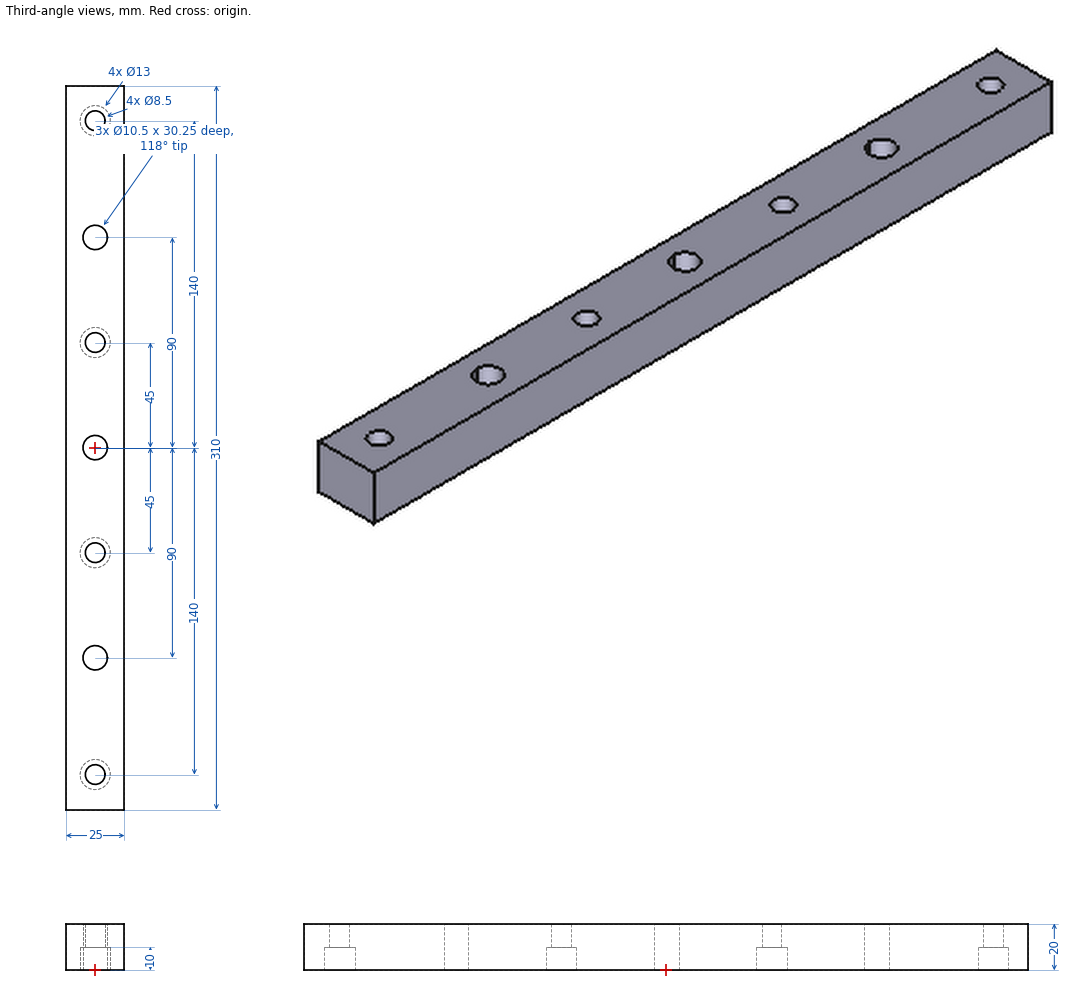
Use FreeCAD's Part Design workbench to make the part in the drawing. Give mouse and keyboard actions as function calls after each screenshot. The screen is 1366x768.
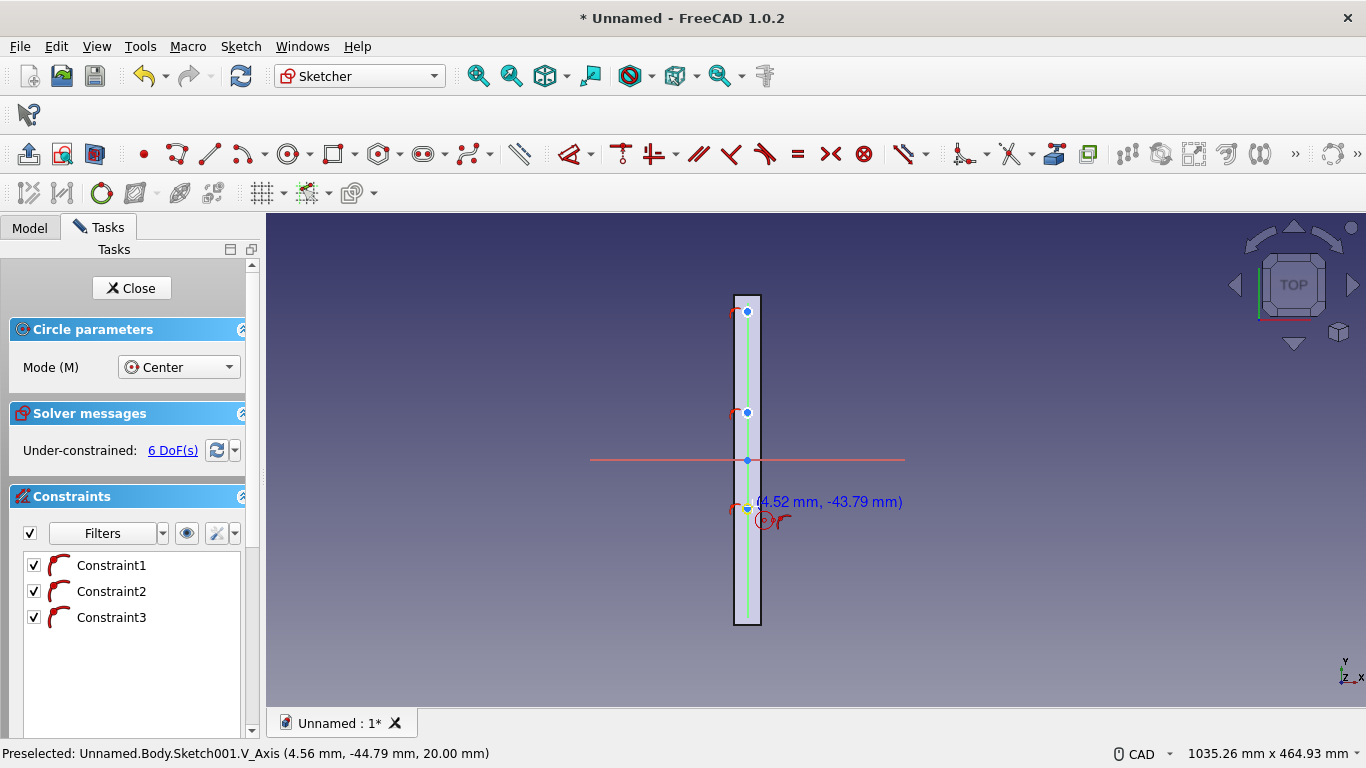
scroll(748, 609, up, 9)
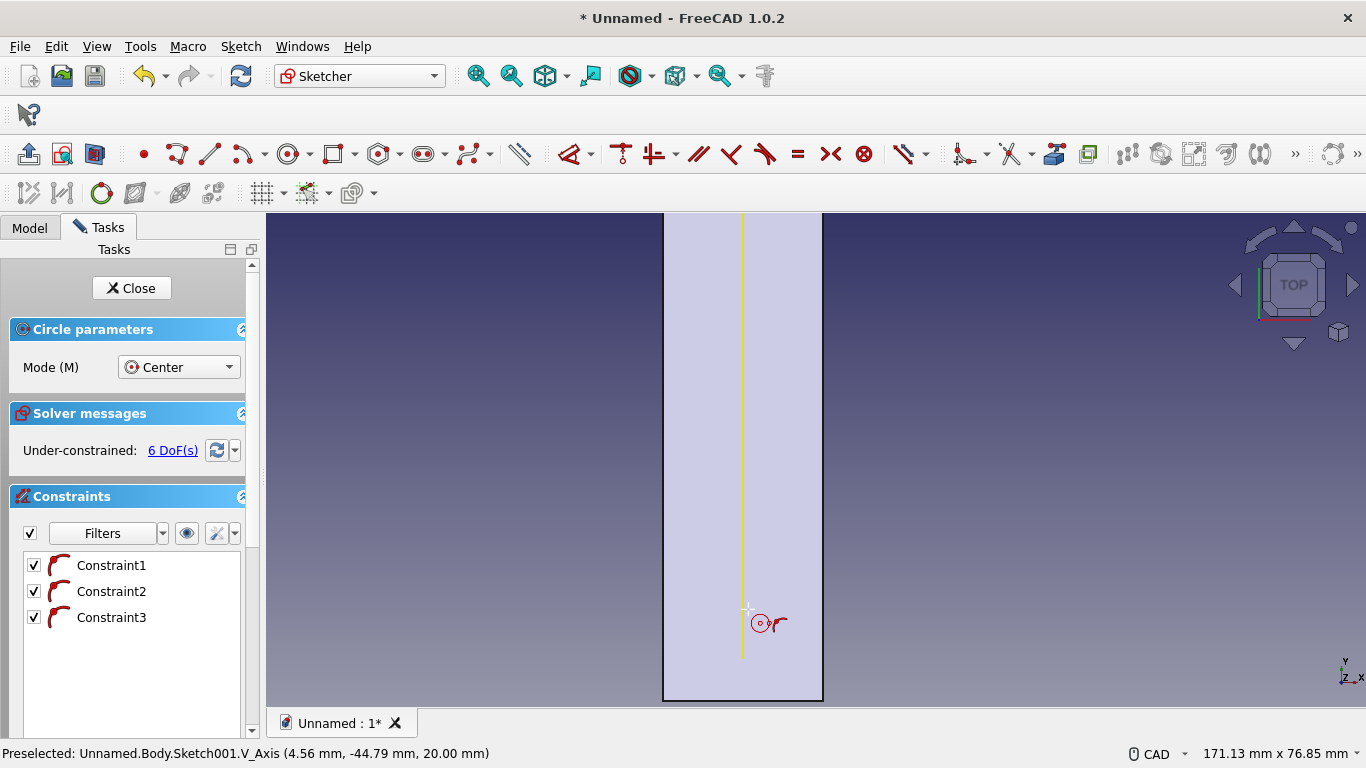
scroll(748, 610, down, 9)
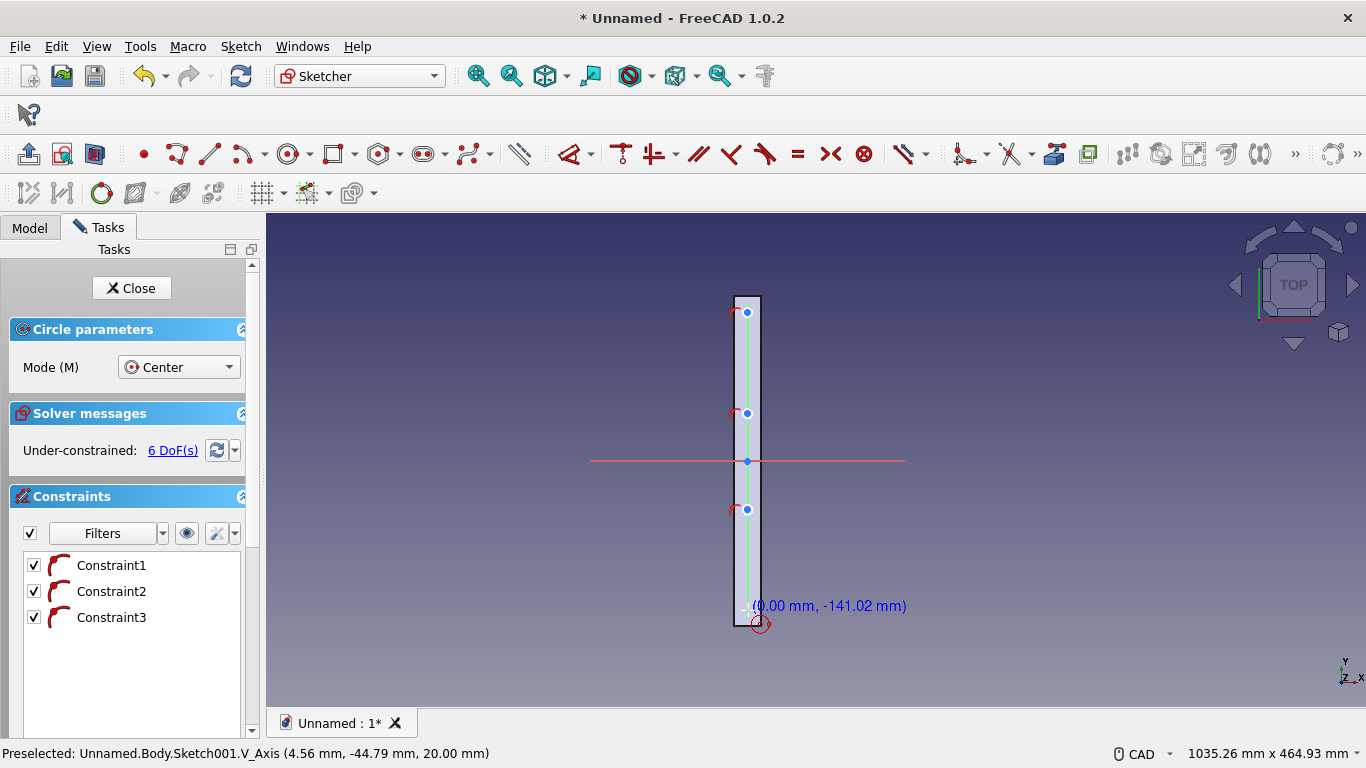
click(748, 610)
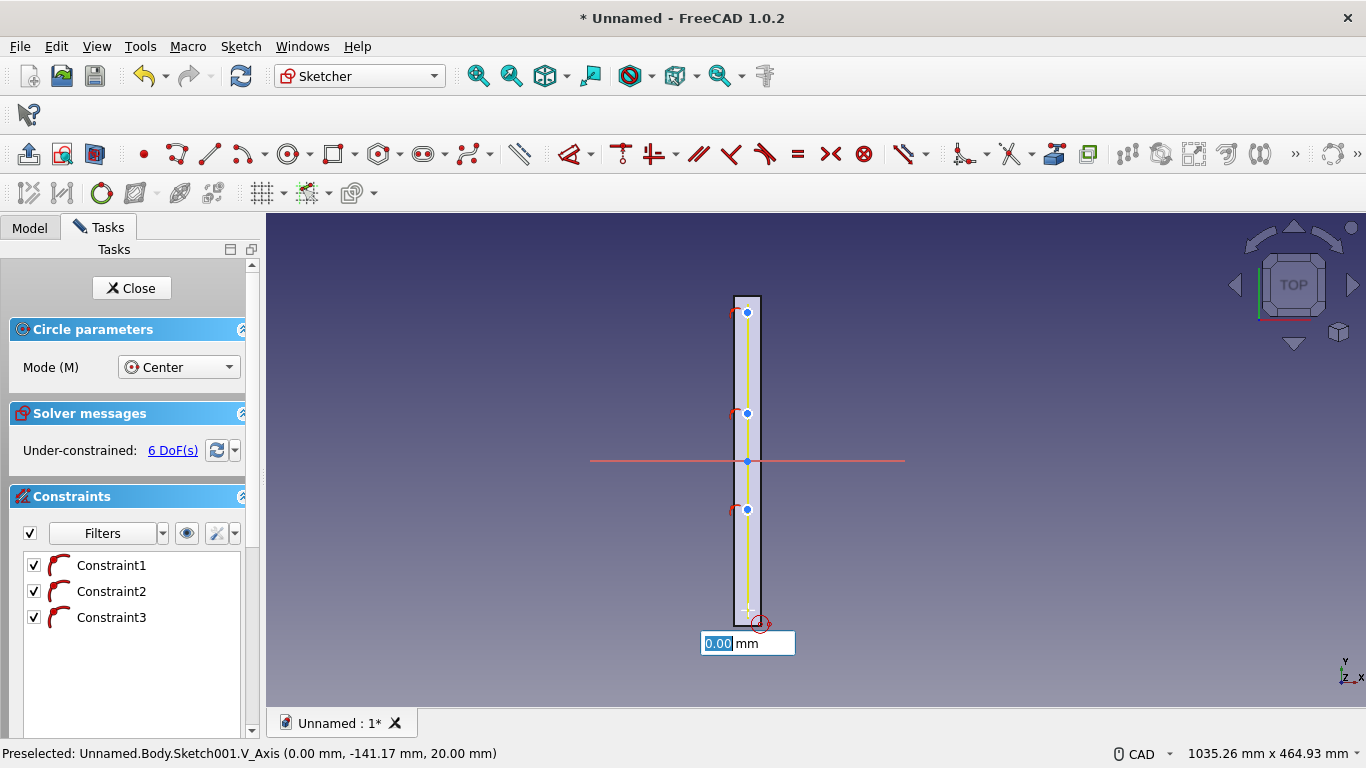
scroll(752, 608, up, 7)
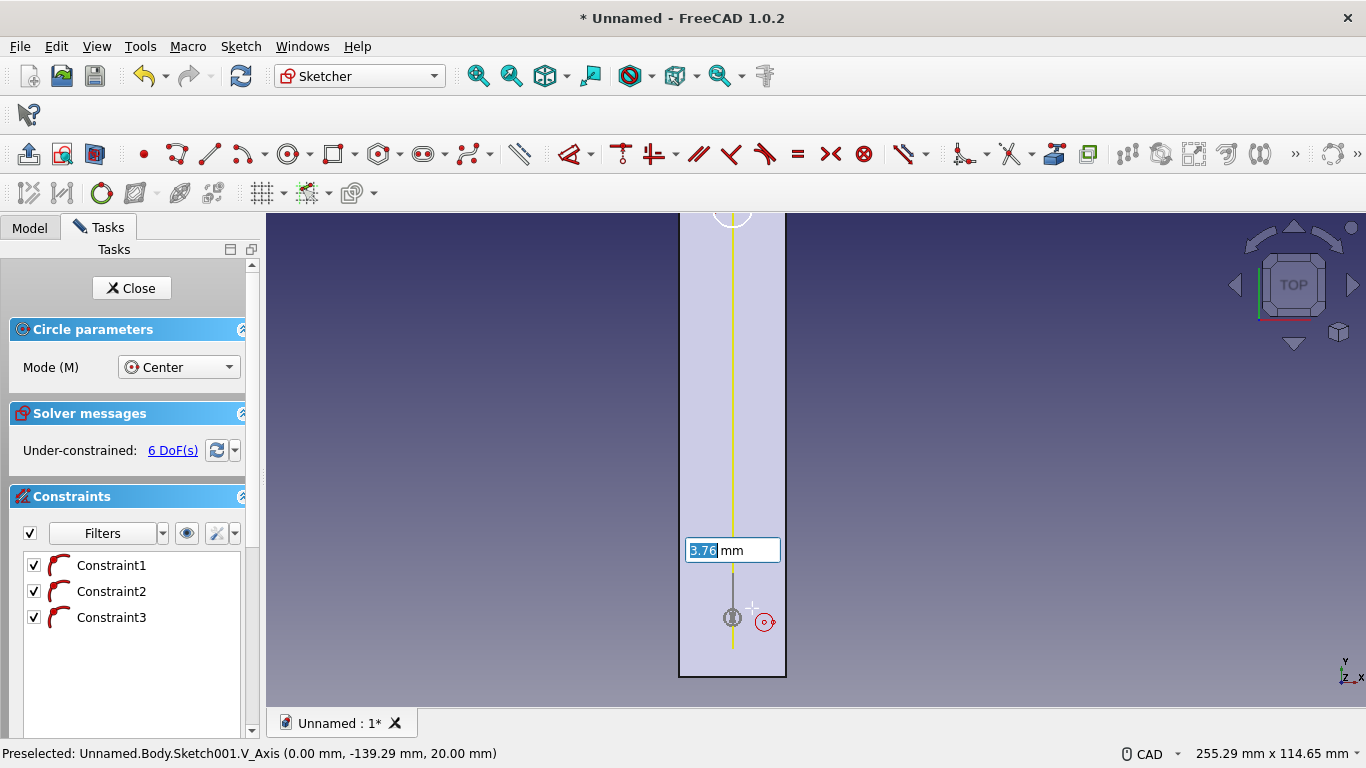
click(750, 606)
key(Escape)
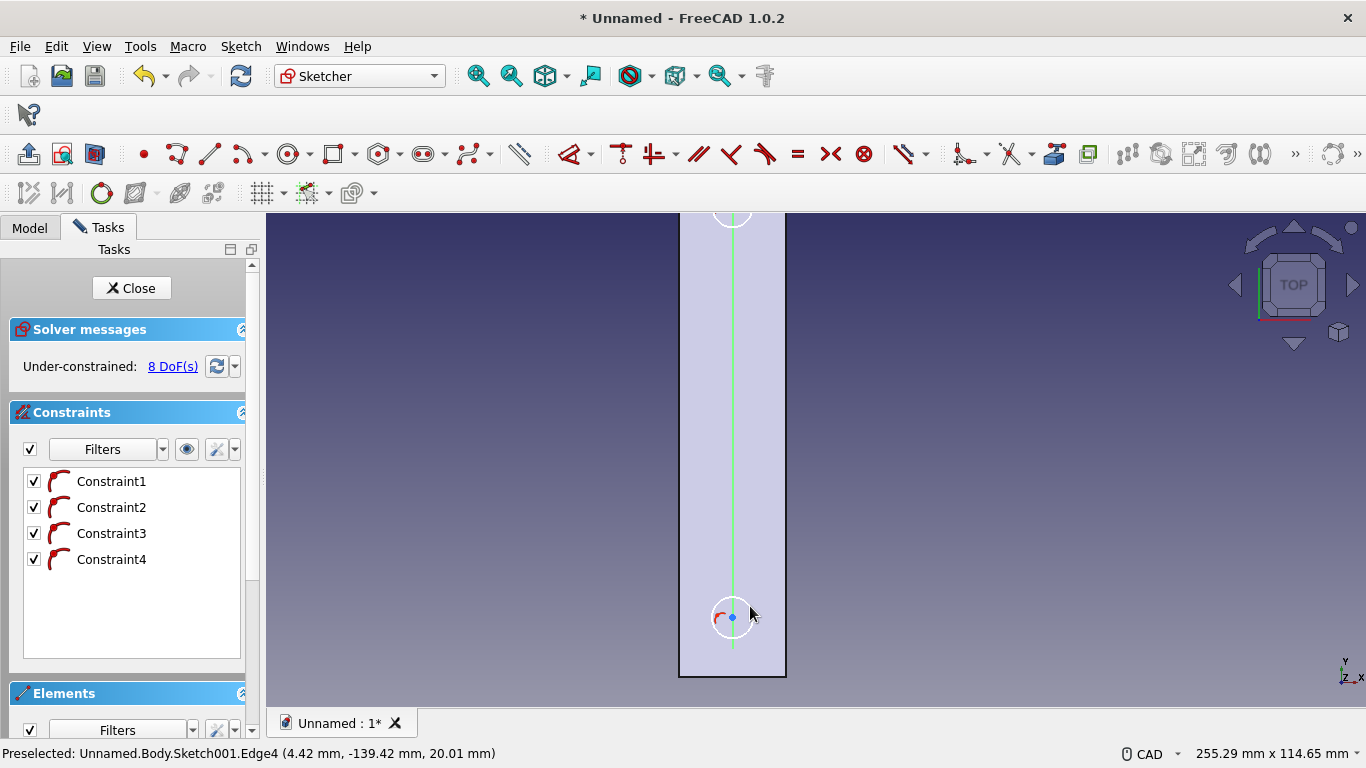
scroll(752, 607, down, 7)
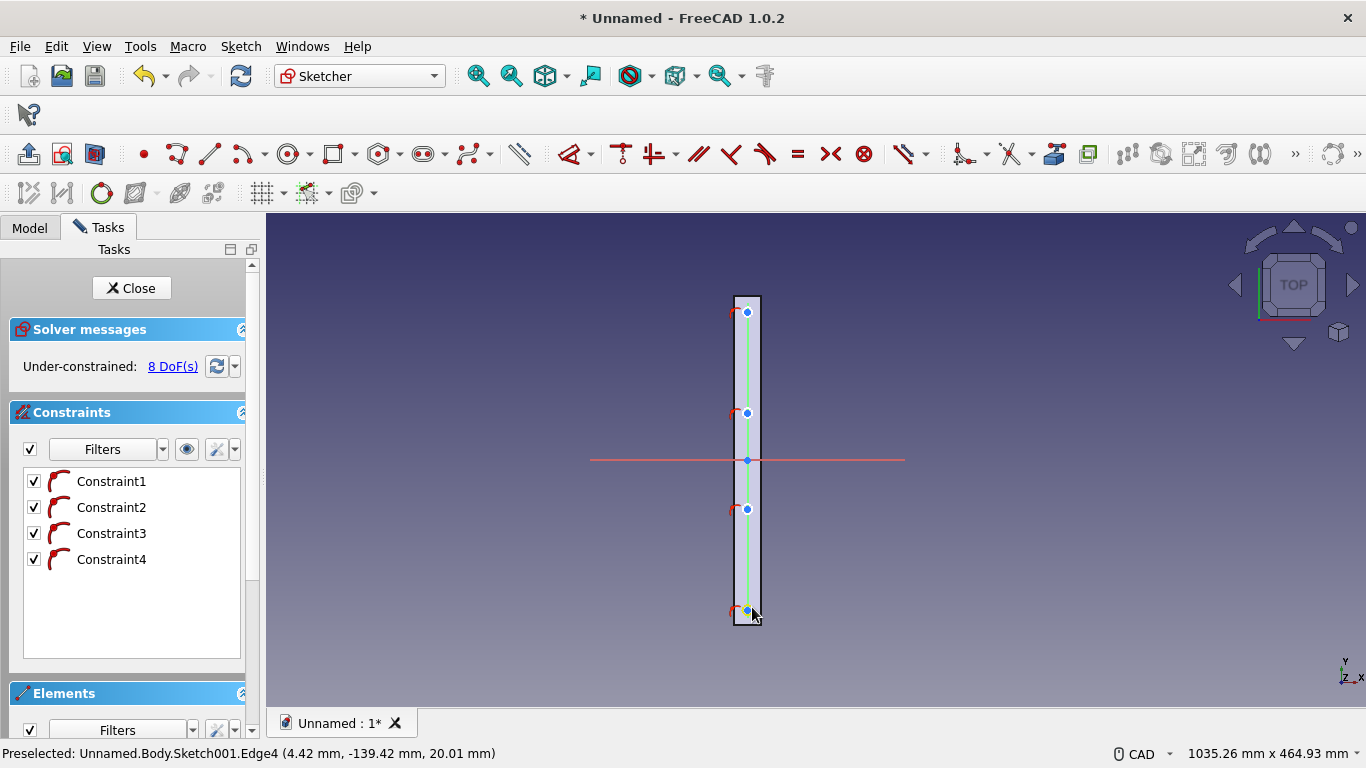
scroll(751, 309, up, 8)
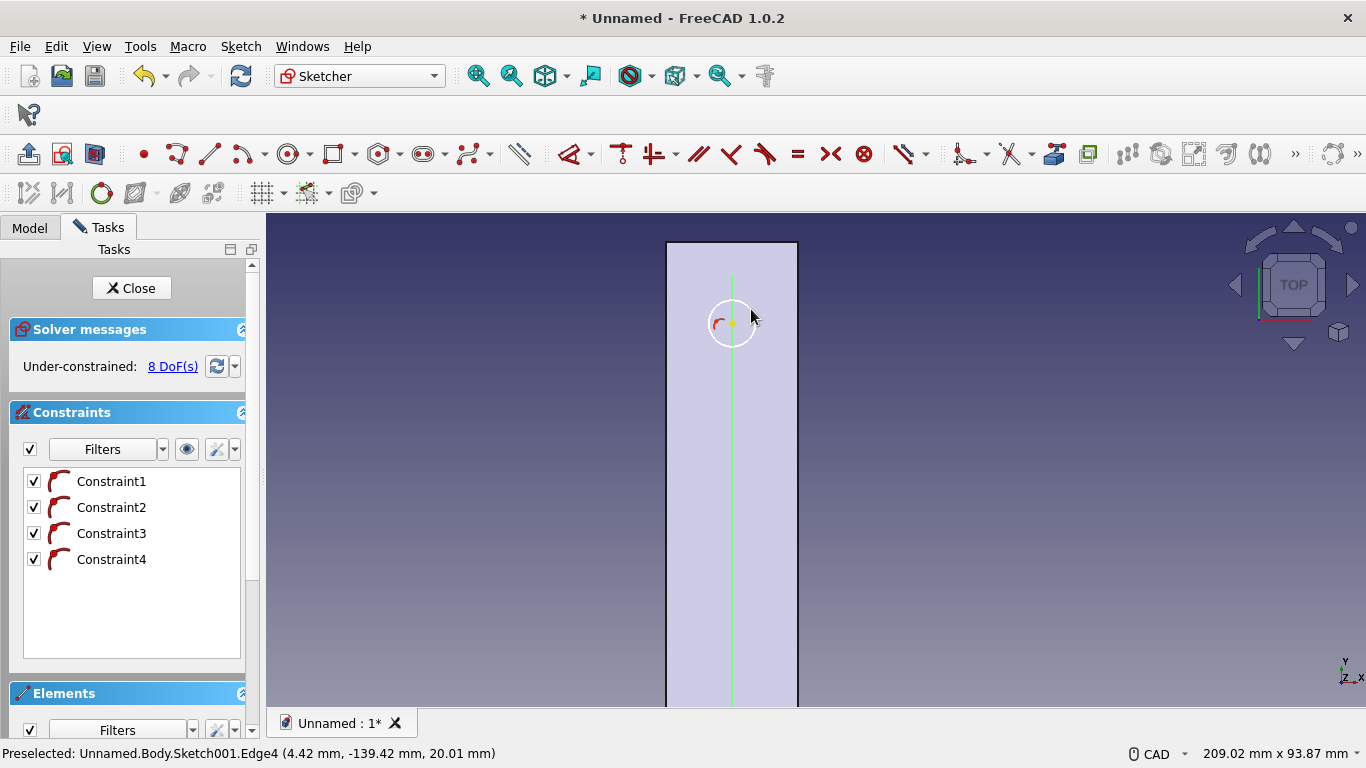
click(748, 307)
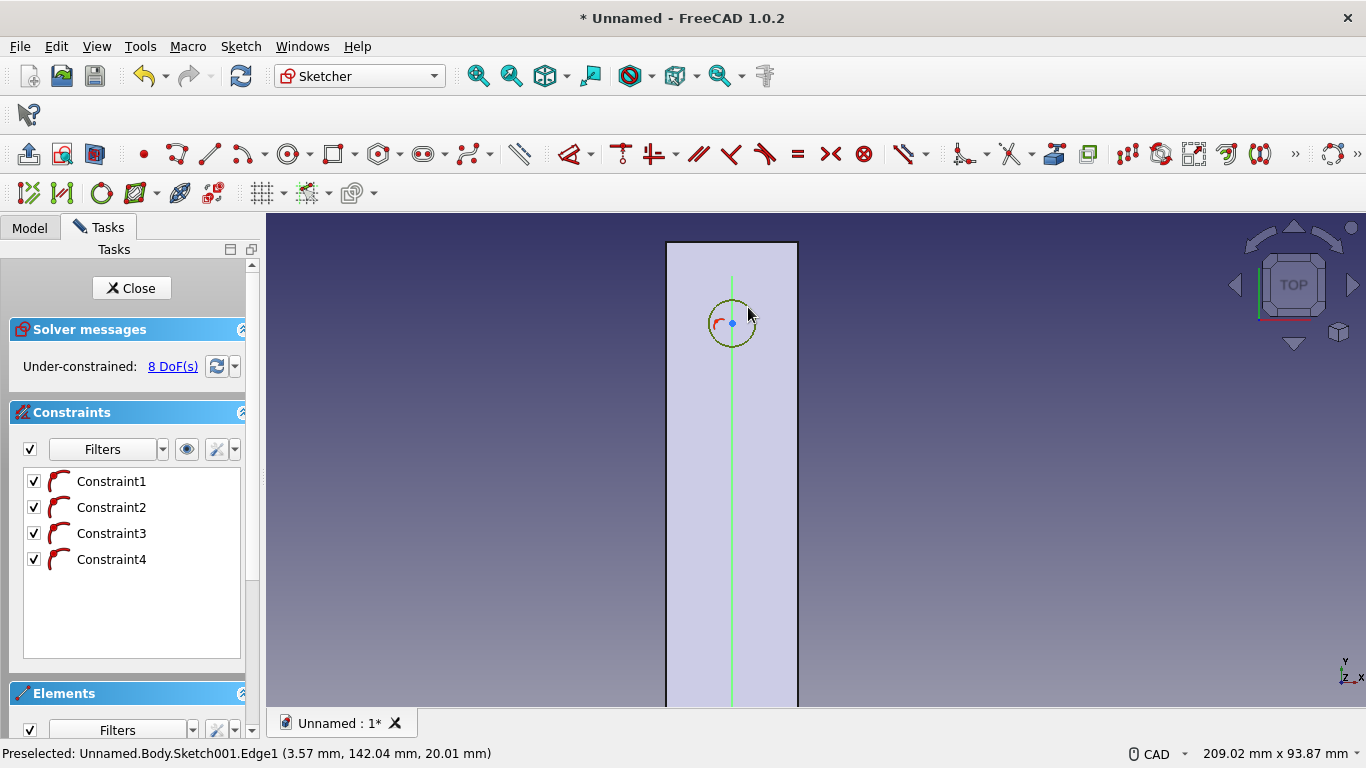
scroll(751, 309, down, 8)